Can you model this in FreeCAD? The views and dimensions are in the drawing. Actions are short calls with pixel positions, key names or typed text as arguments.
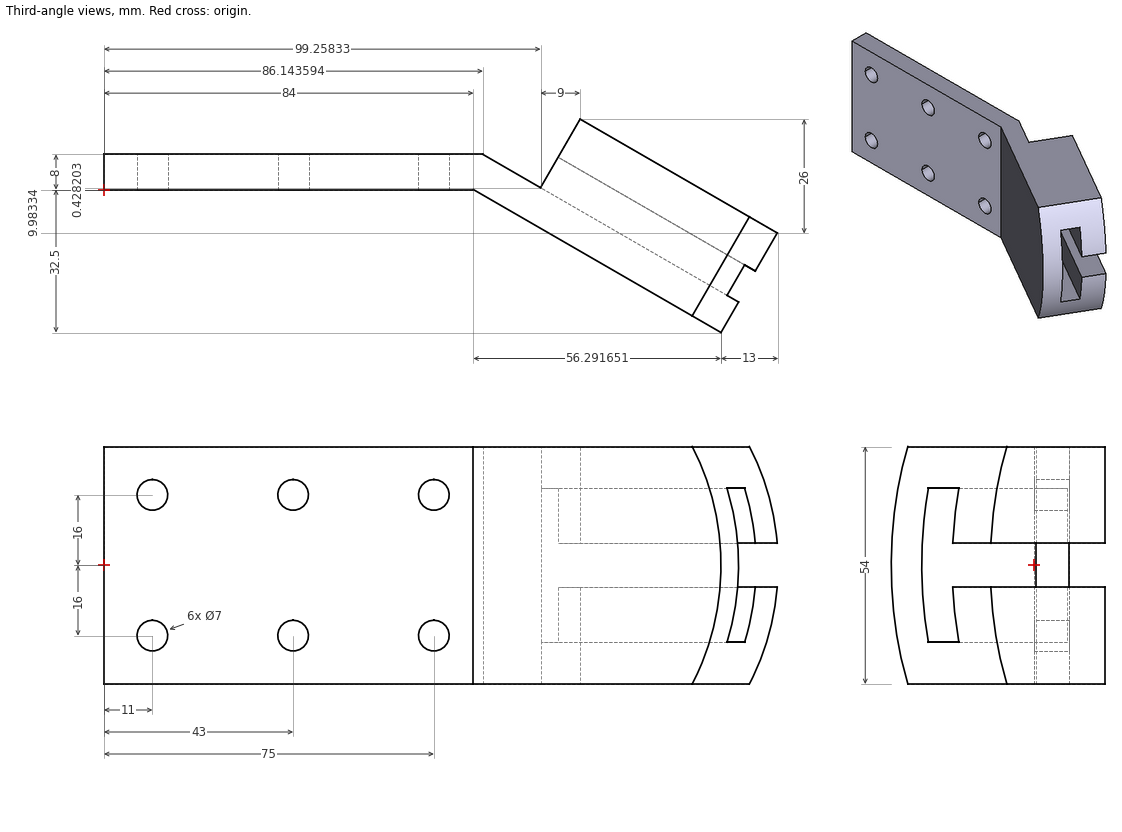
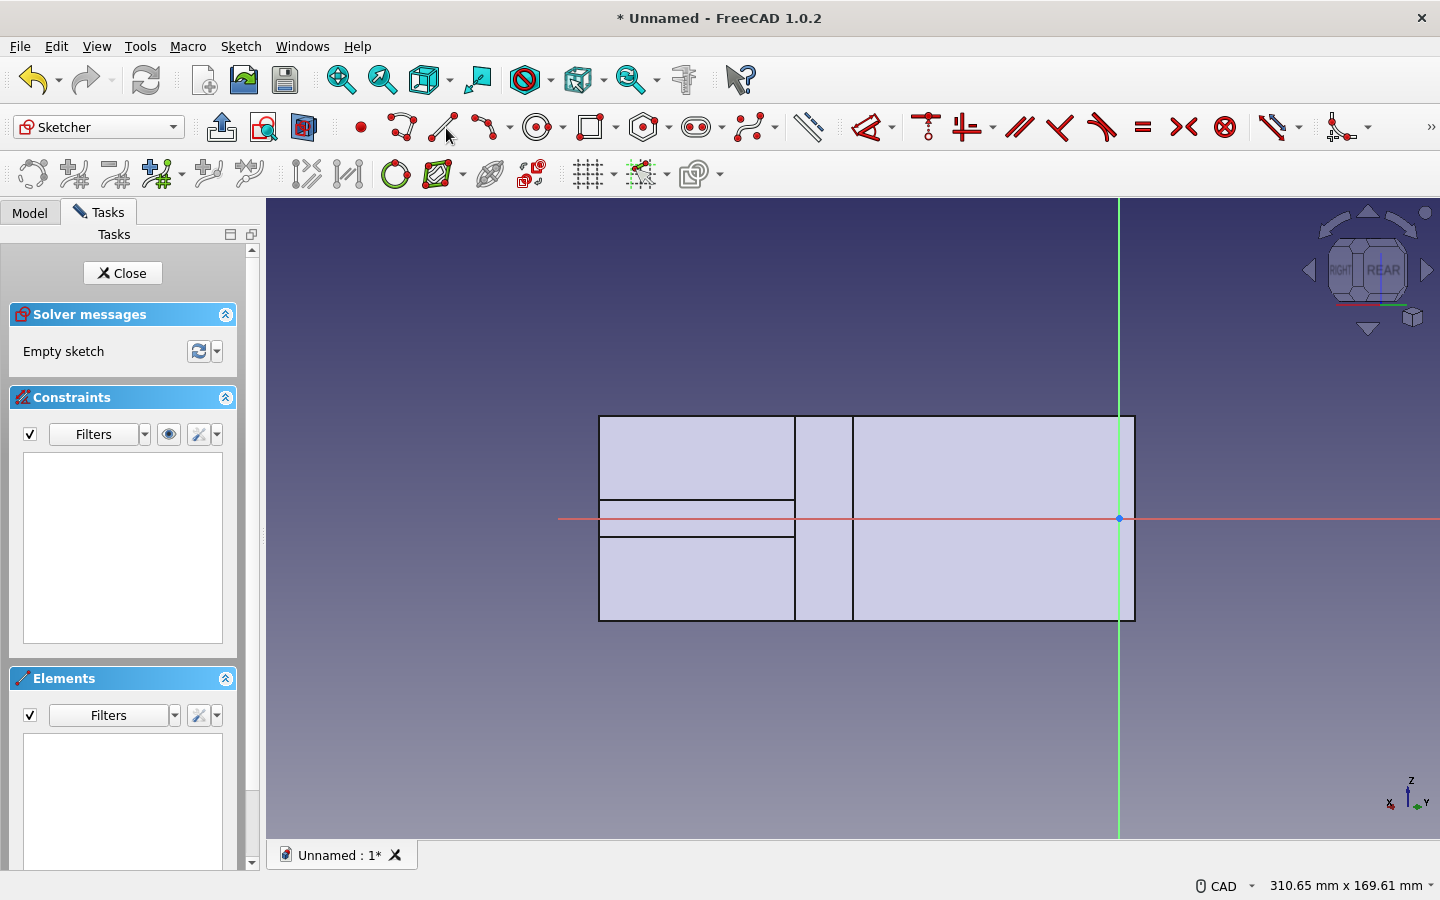
scroll(305, 518, up, 4)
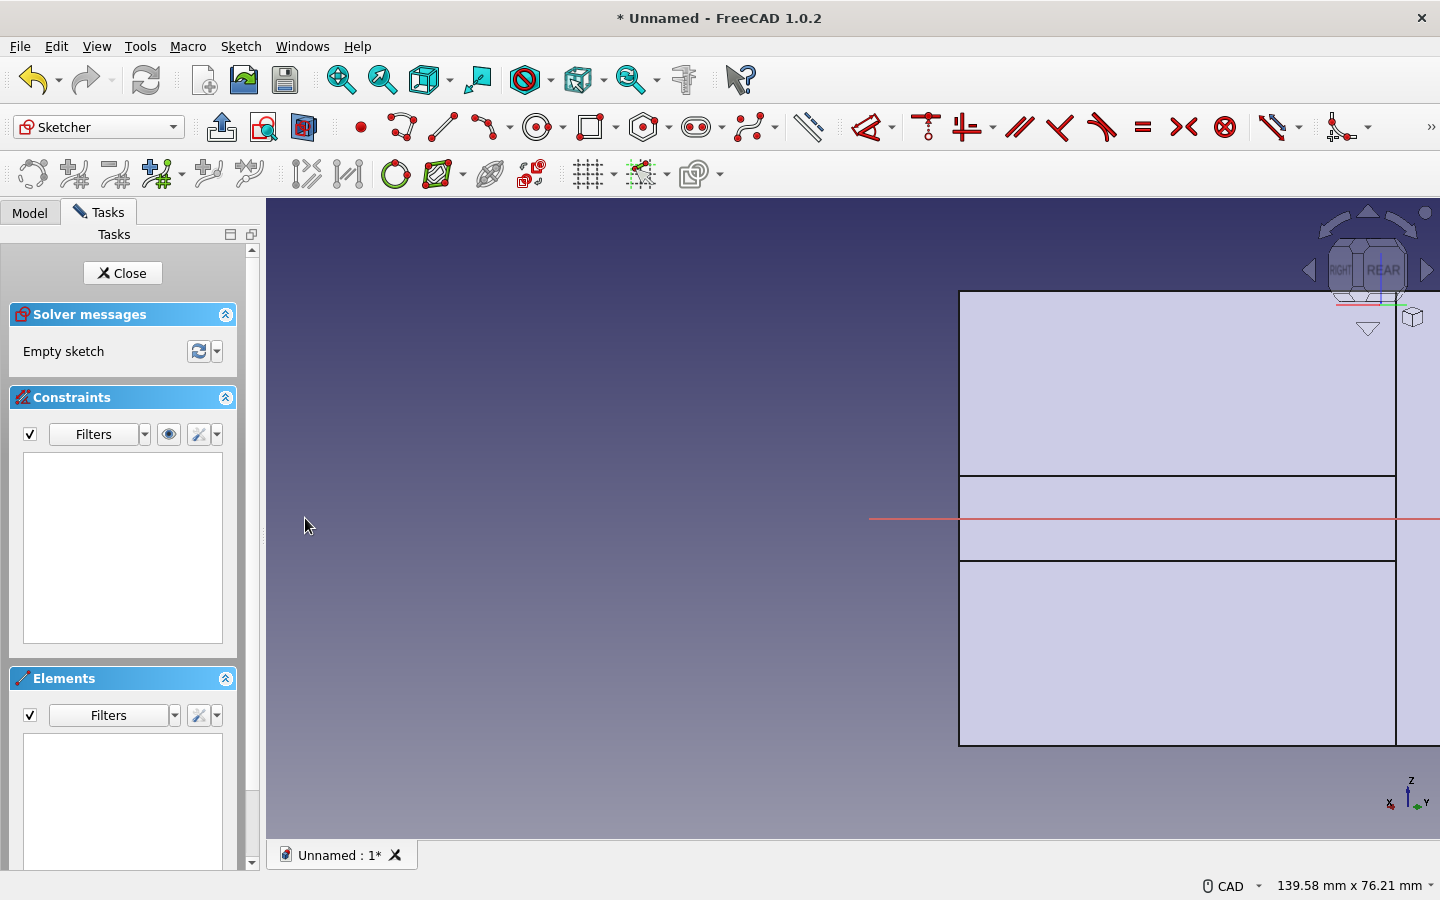
key(g)
key(m)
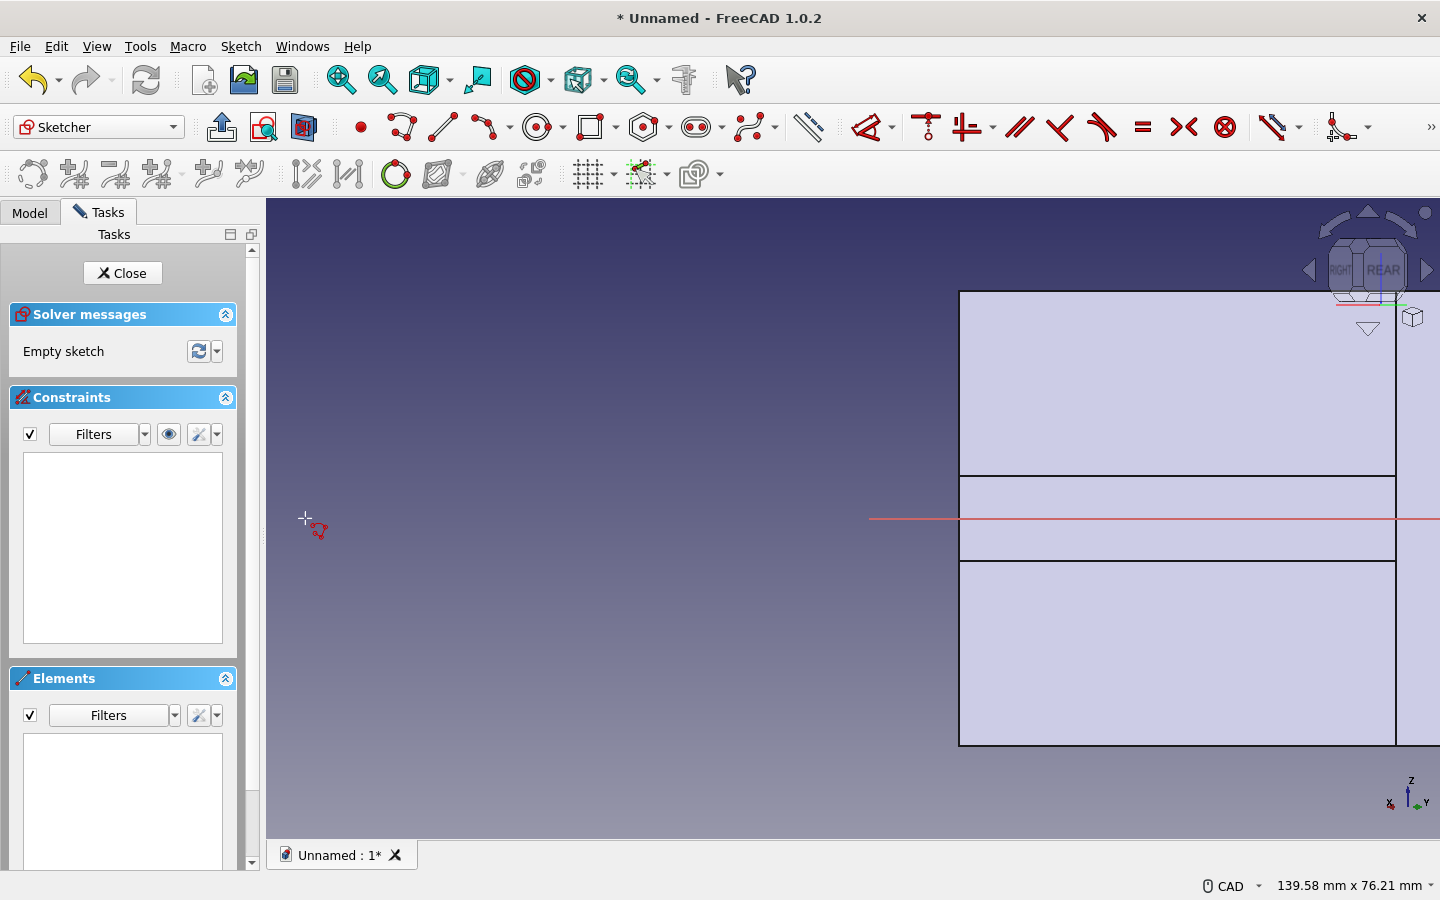
click(1023, 291)
click(547, 291)
click(547, 746)
click(1023, 746)
right_click(1023, 746)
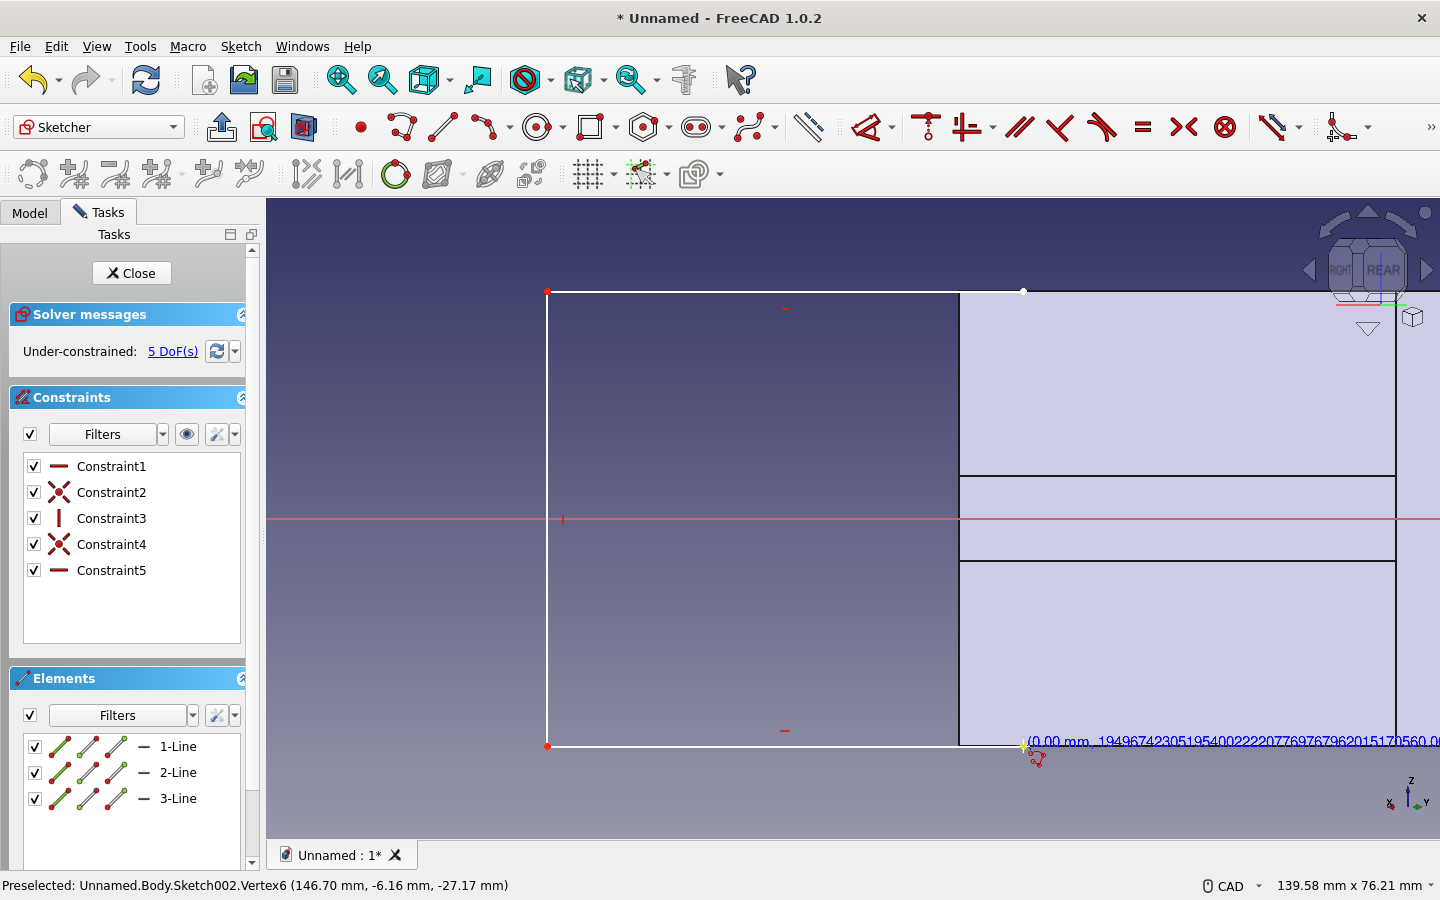
key(g)
key(3)
key(a)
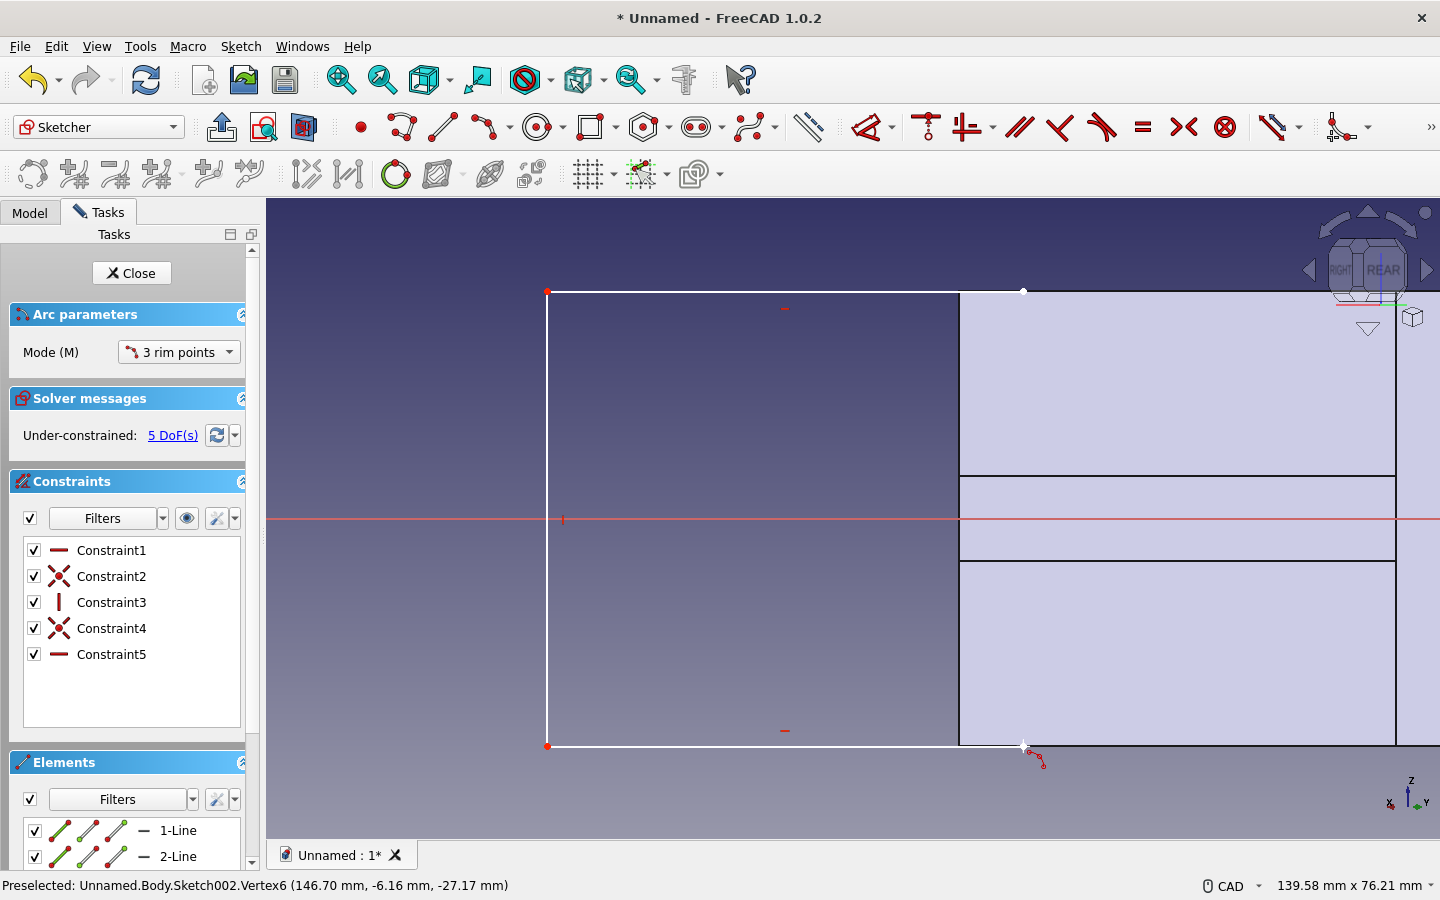
click(1023, 747)
click(1023, 292)
click(962, 471)
key(Escape)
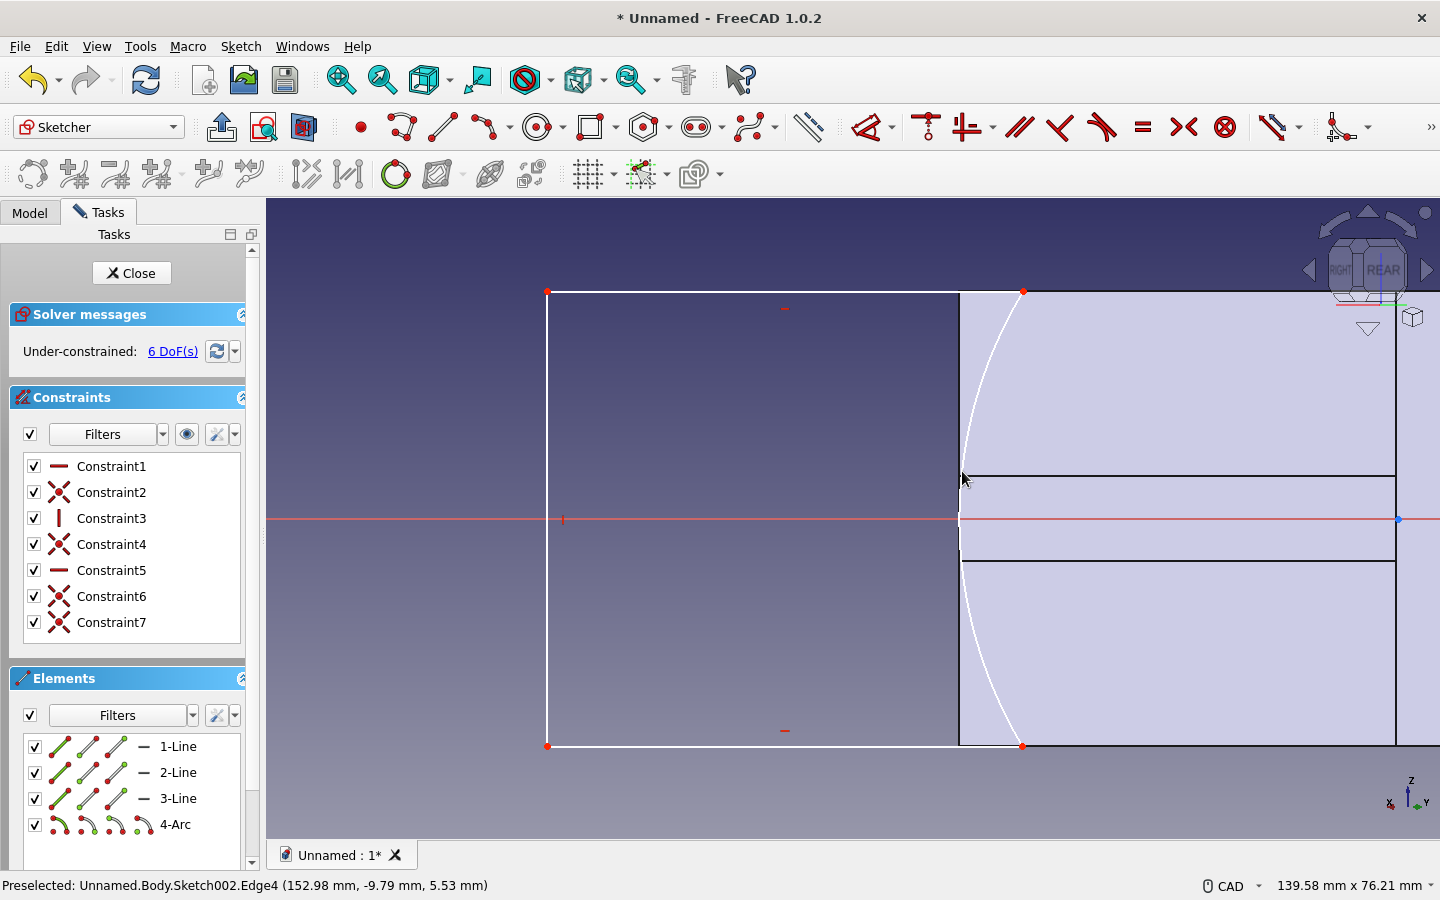
scroll(294, 519, down, 1)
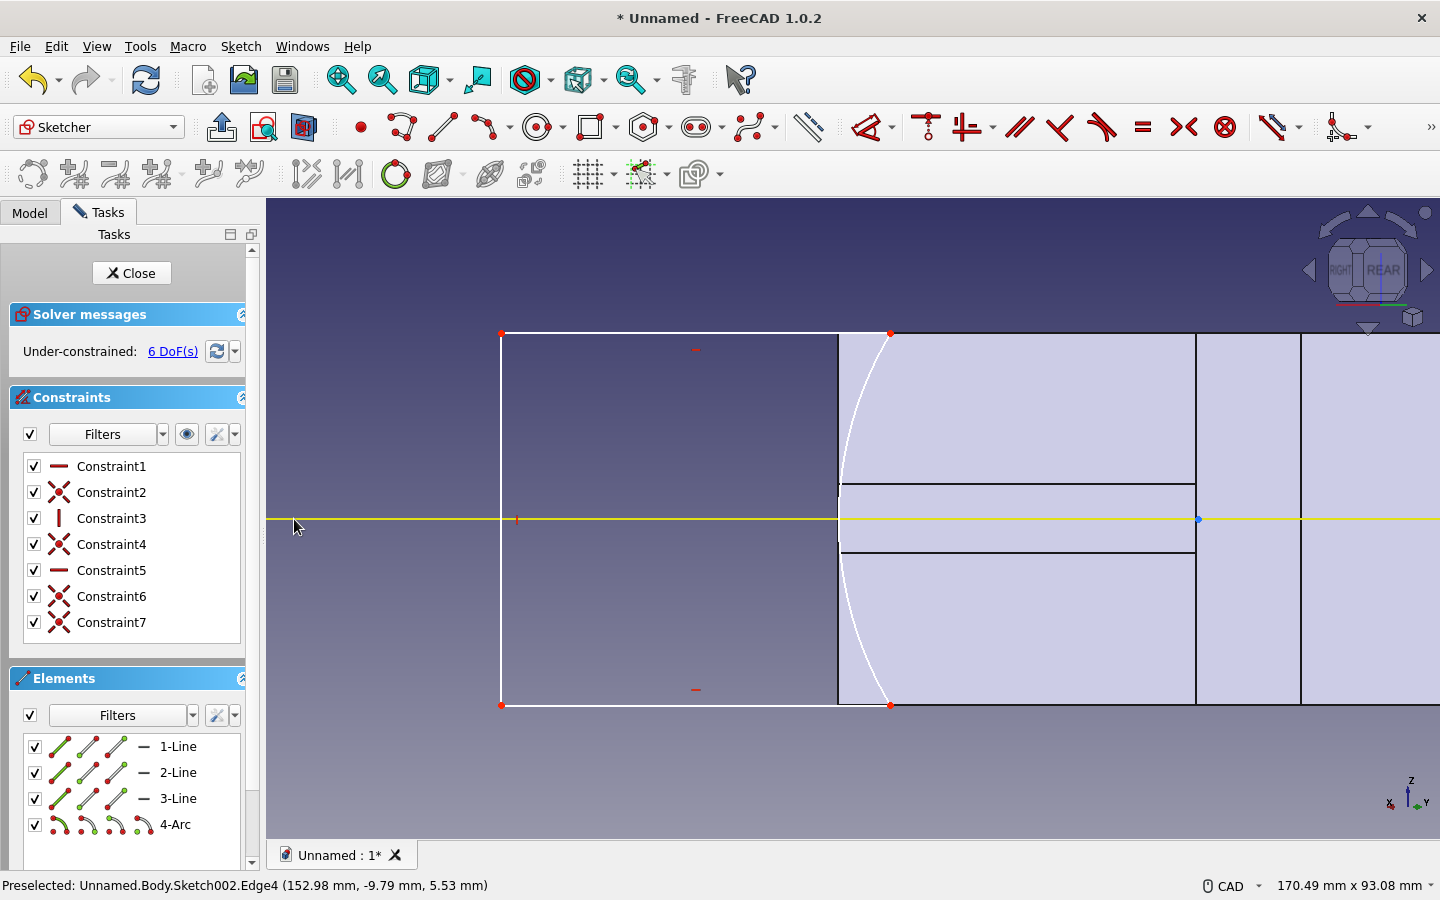
click(1198, 520)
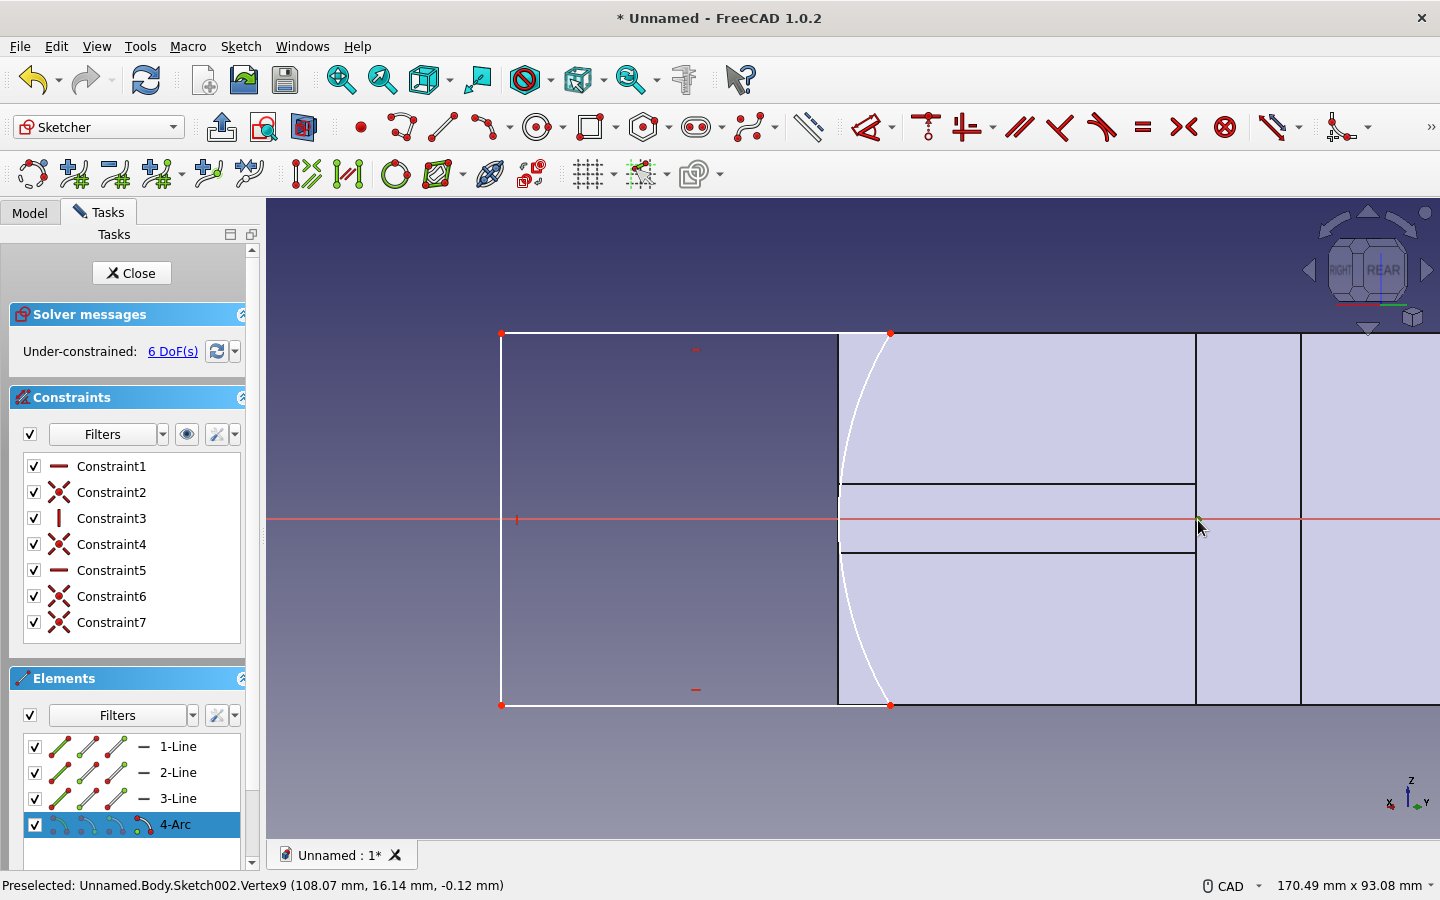
click(364, 519)